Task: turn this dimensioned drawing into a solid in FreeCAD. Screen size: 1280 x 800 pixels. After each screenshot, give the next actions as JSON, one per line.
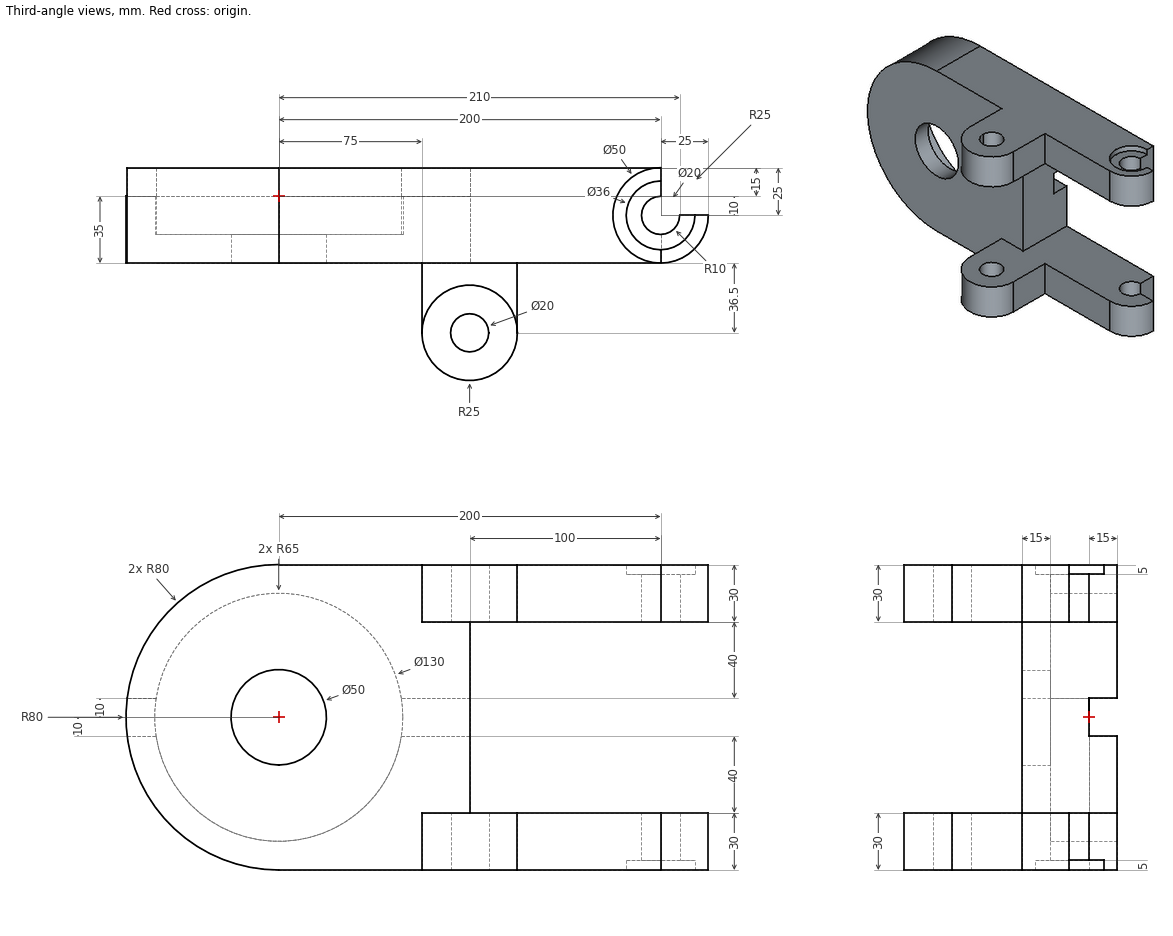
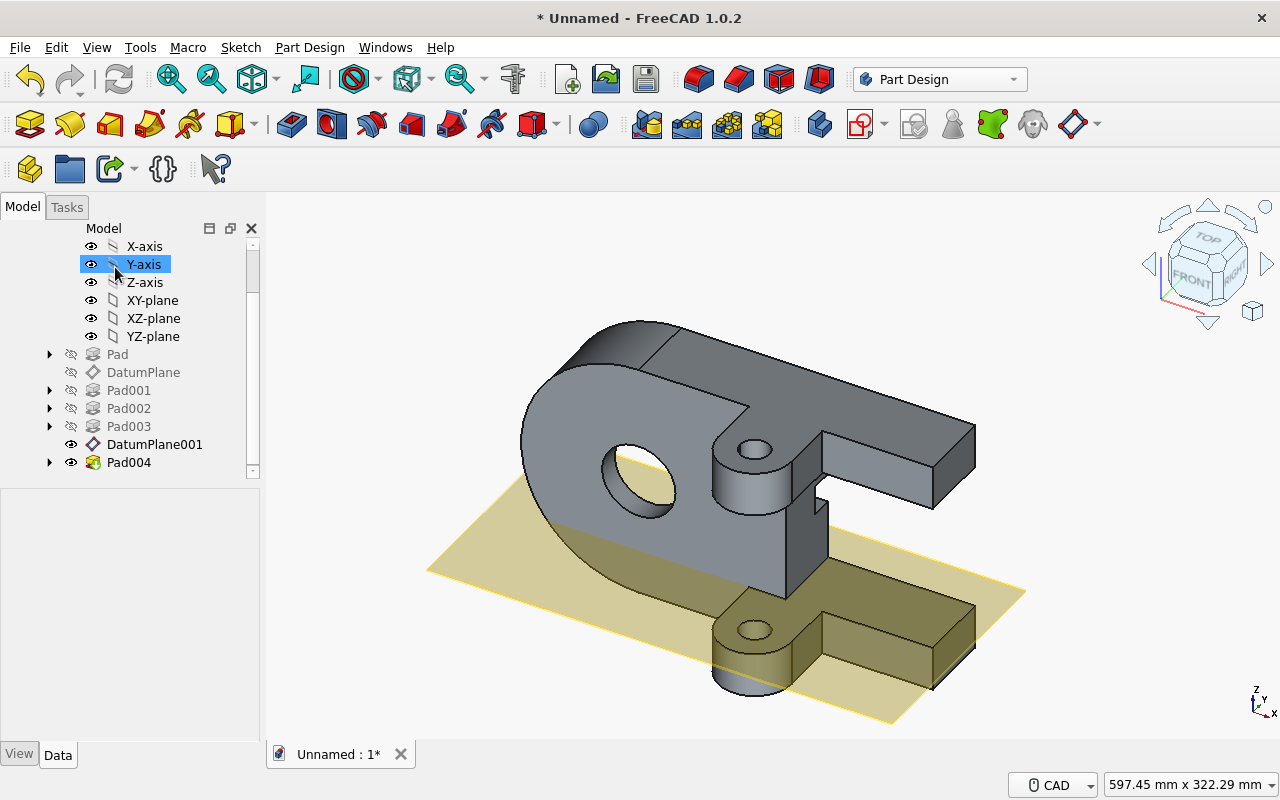
{"action": "left_click", "coordinate": [116, 444]}
{"action": "key", "text": "space"}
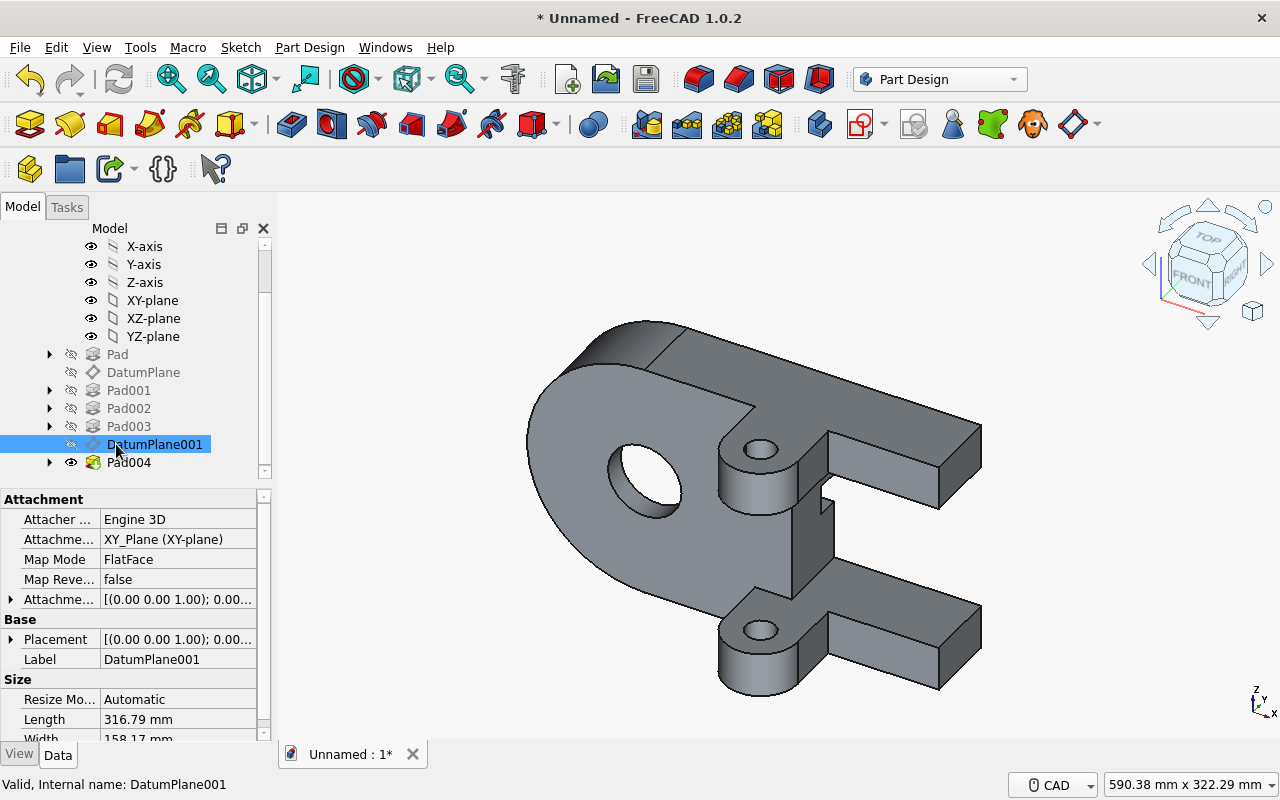
{"action": "left_click", "coordinate": [172, 80]}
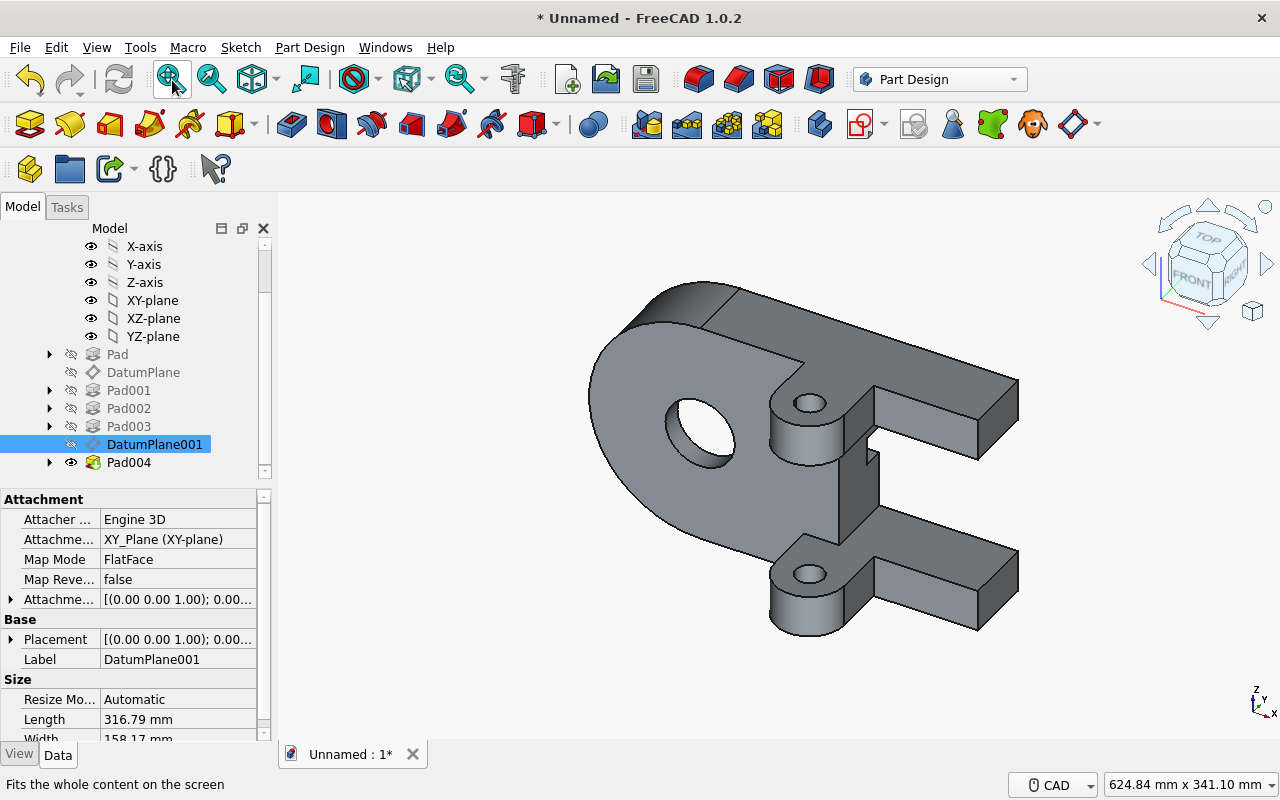
{"action": "left_click", "coordinate": [847, 365]}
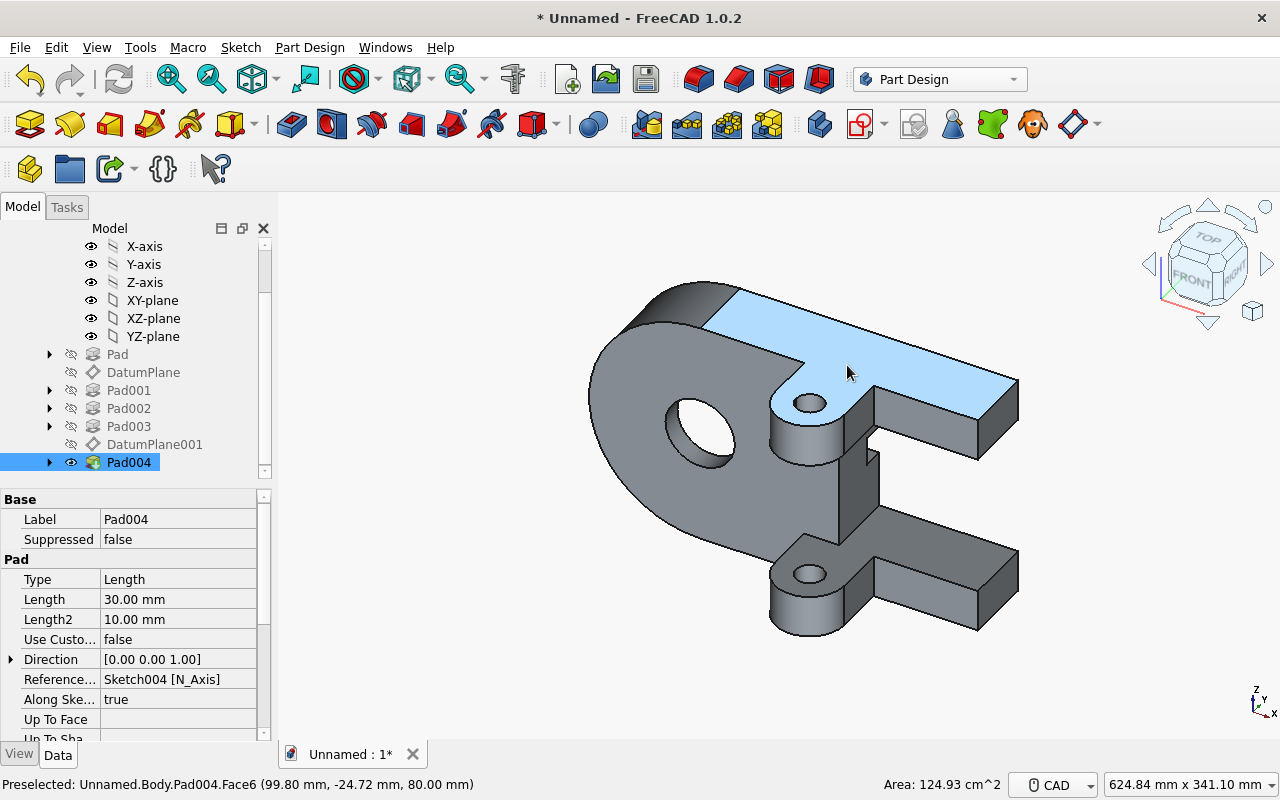
{"action": "left_click", "coordinate": [860, 124]}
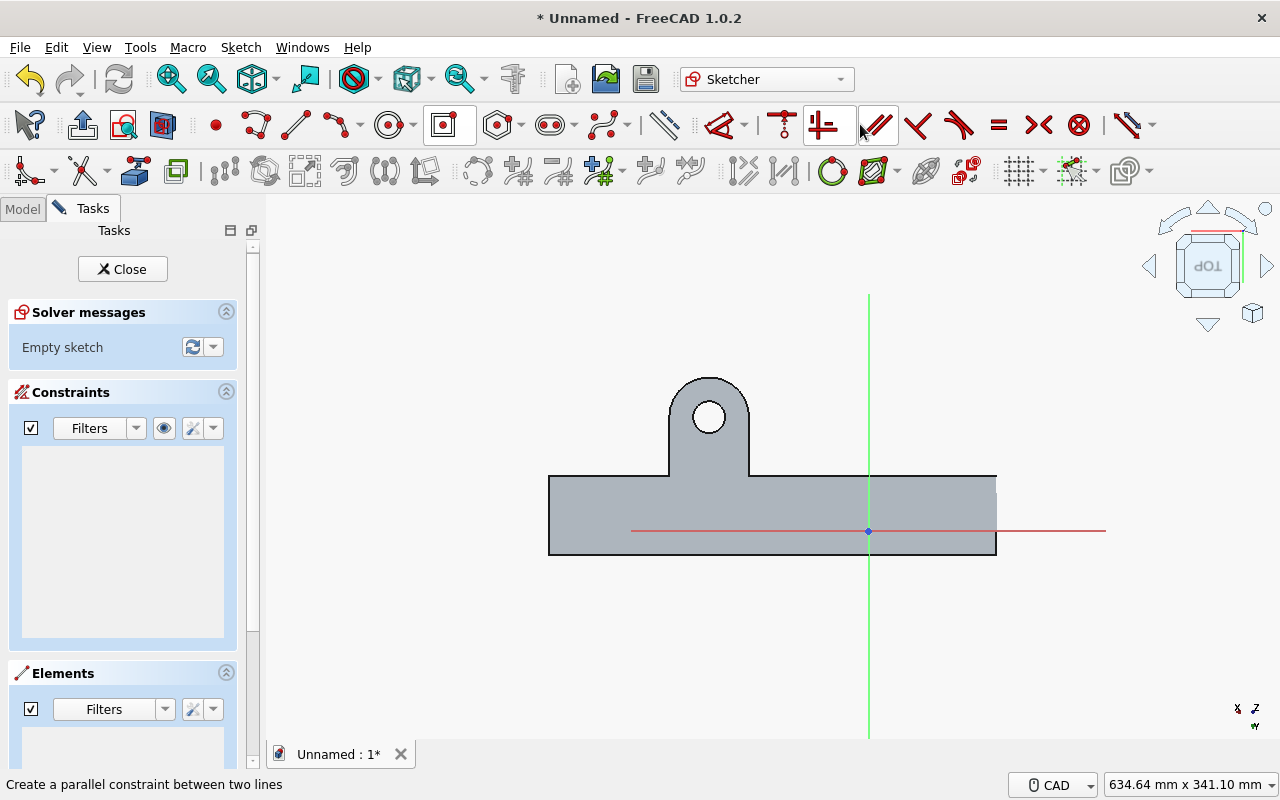
{"action": "scroll", "coordinate": [499, 532], "scroll_direction": "up", "scroll_amount": 7}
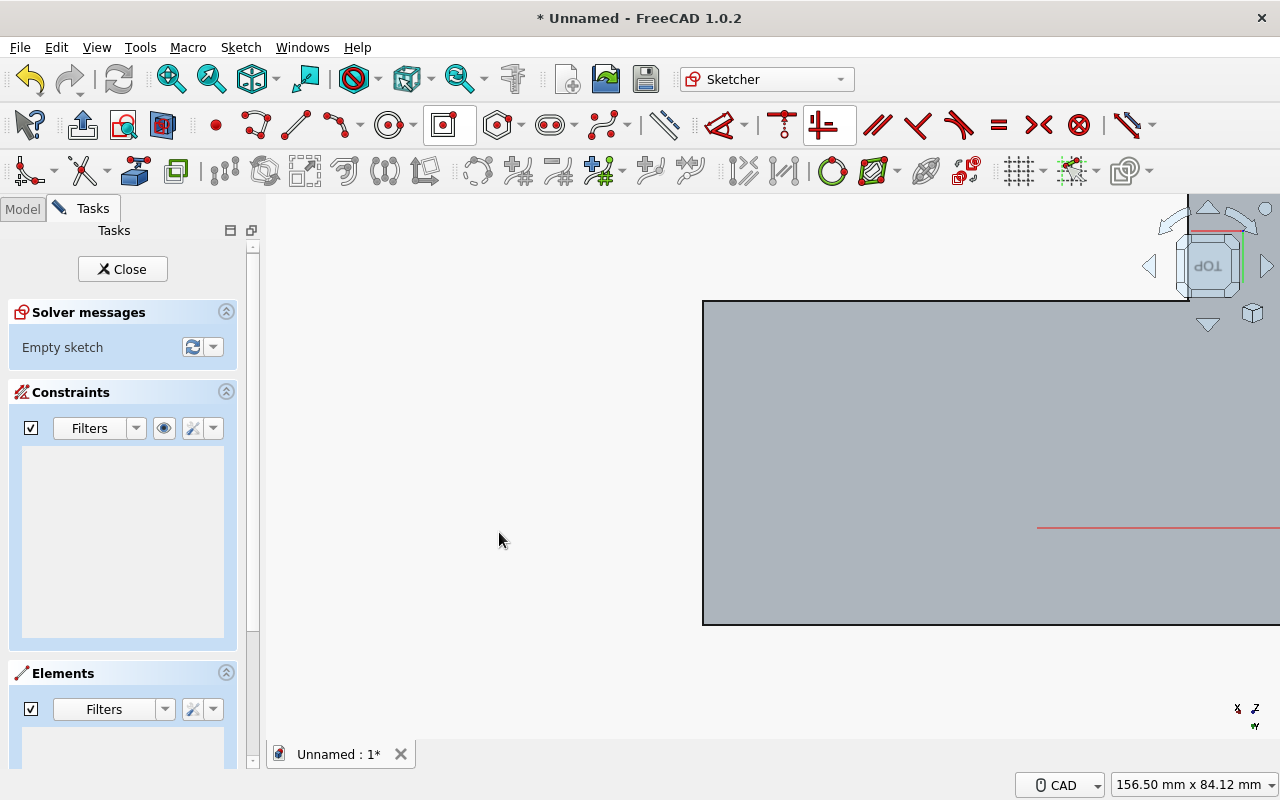
{"action": "left_click", "coordinate": [390, 126]}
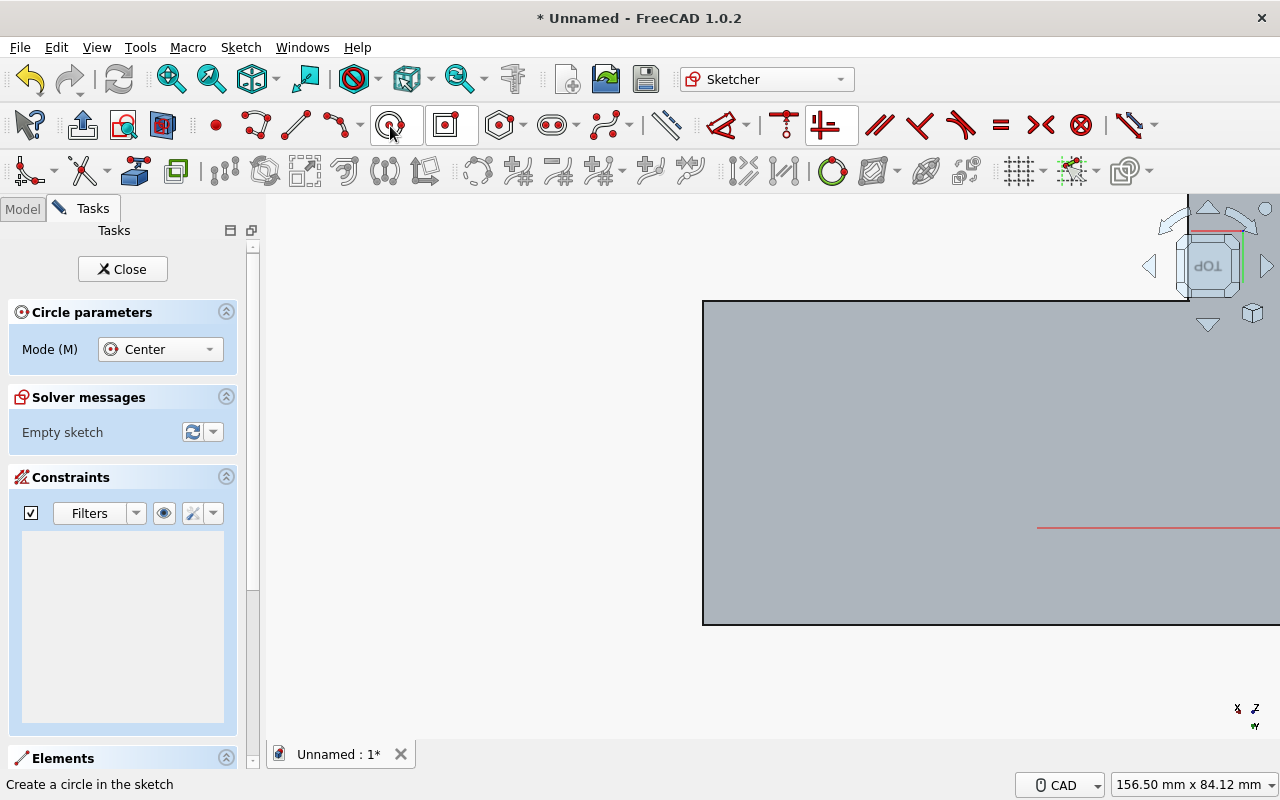
{"action": "left_click", "coordinate": [703, 463]}
{"action": "left_click", "coordinate": [817, 349]}
{"action": "key", "text": "Escape"}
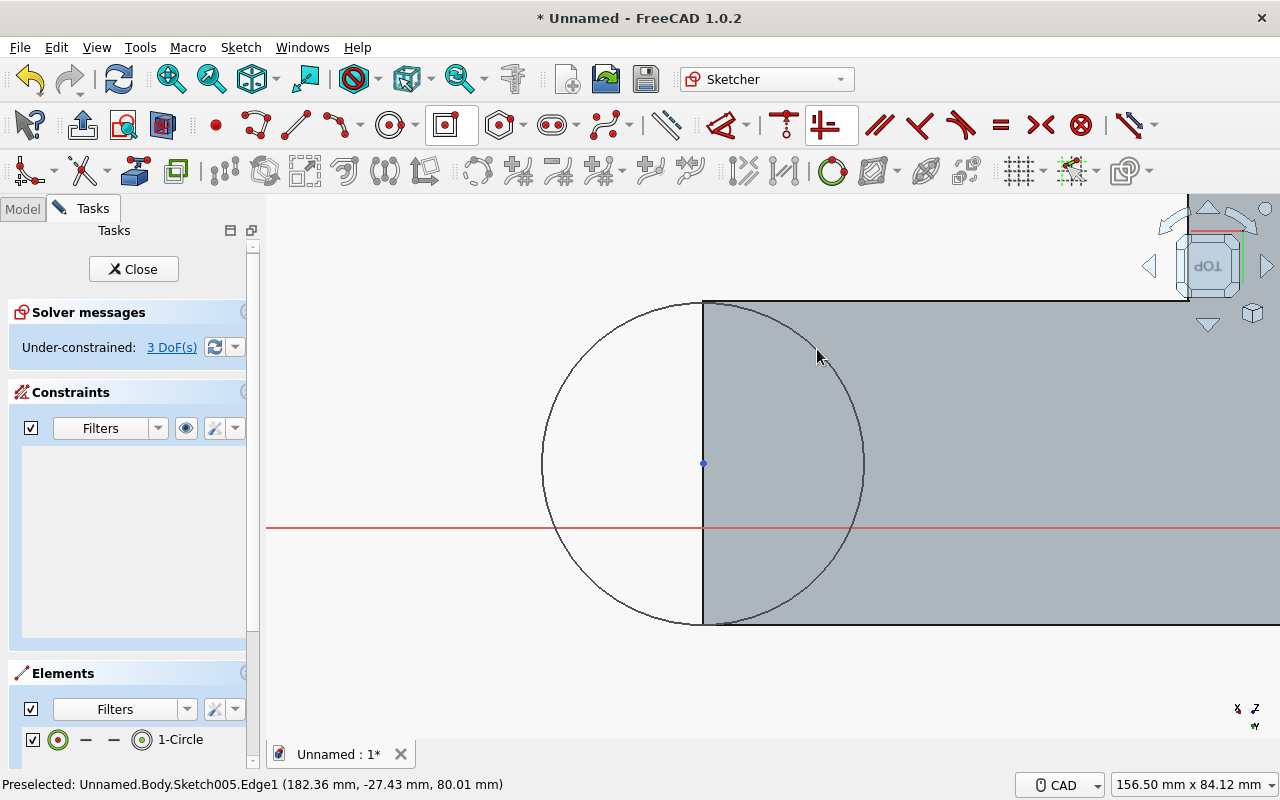
{"action": "left_click", "coordinate": [722, 126]}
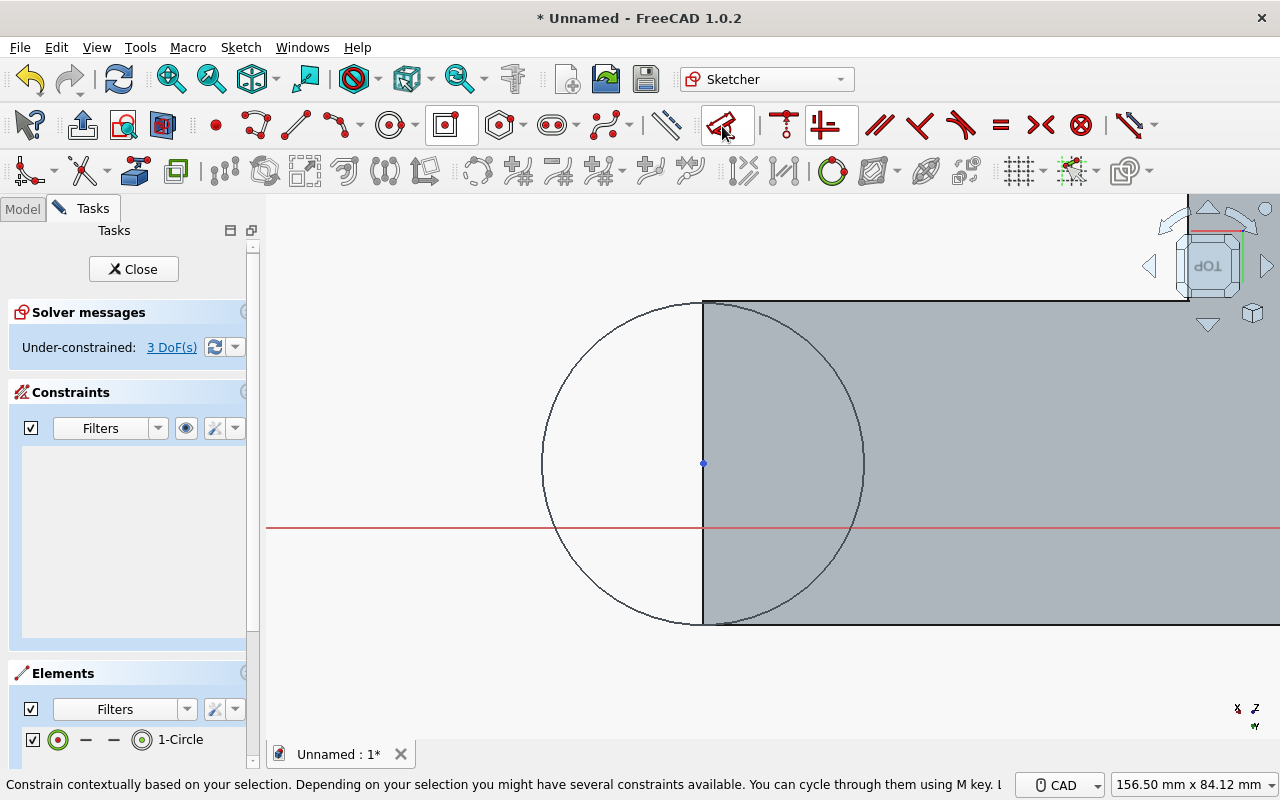
{"action": "left_click", "coordinate": [817, 350]}
{"action": "left_click", "coordinate": [840, 327]}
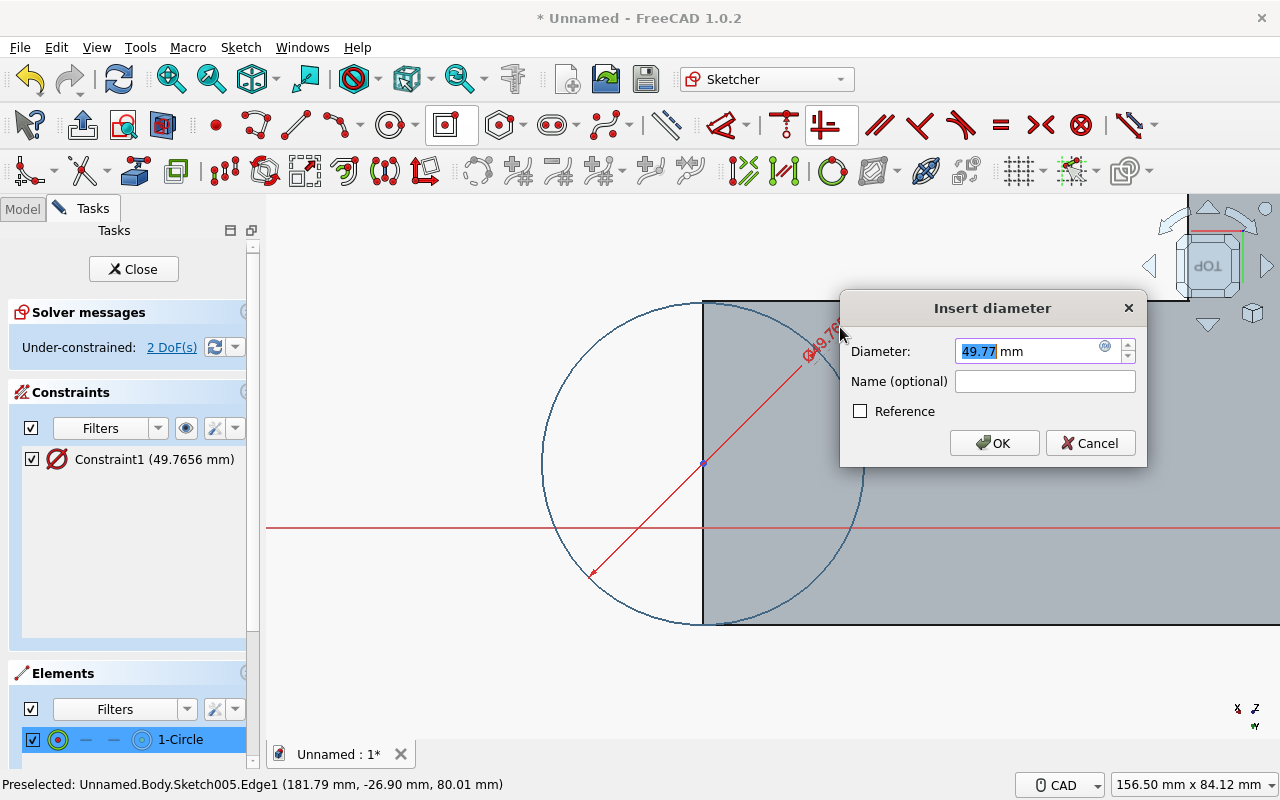
{"action": "type", "text": "50"}
{"action": "key", "text": "Return"}